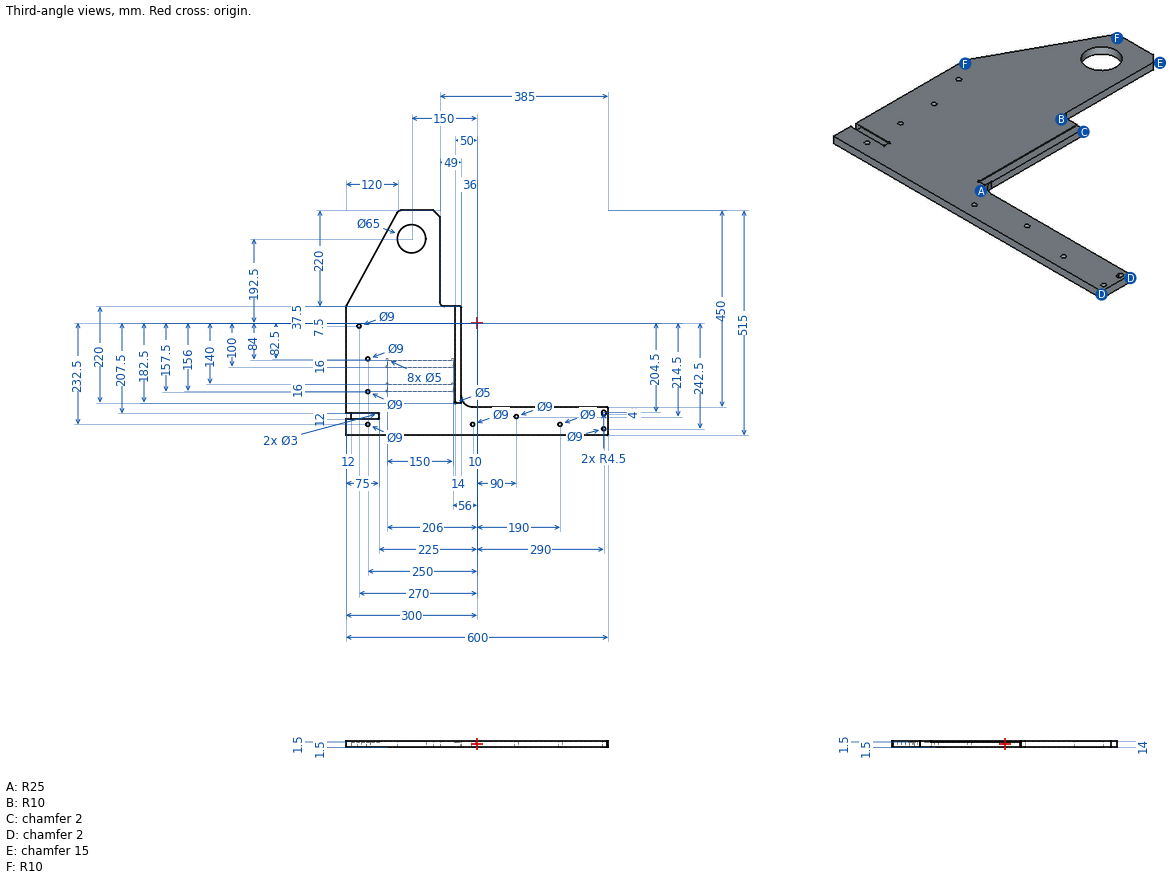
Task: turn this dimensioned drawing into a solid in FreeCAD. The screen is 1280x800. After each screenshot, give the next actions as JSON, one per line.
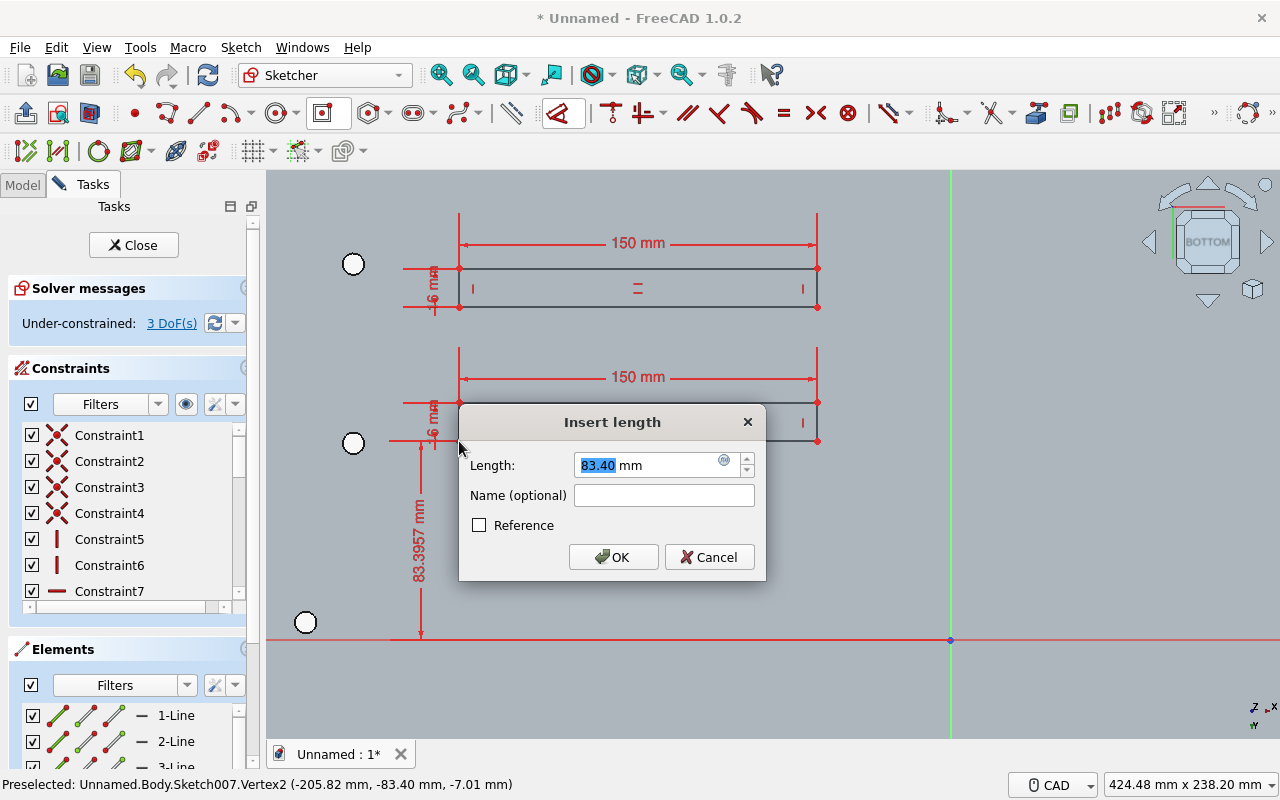
{"action": "type", "text": "84"}
{"action": "key", "text": "Return"}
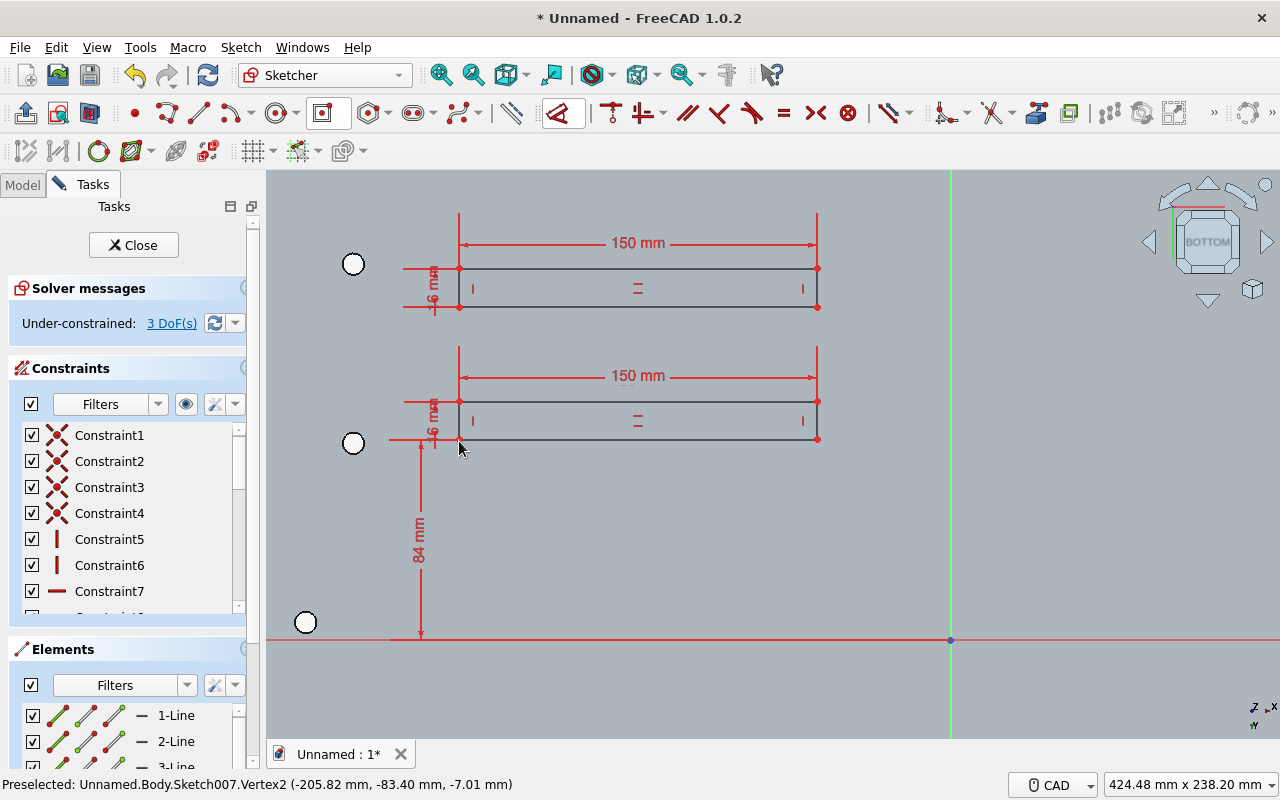
{"action": "left_click", "coordinate": [817, 440]}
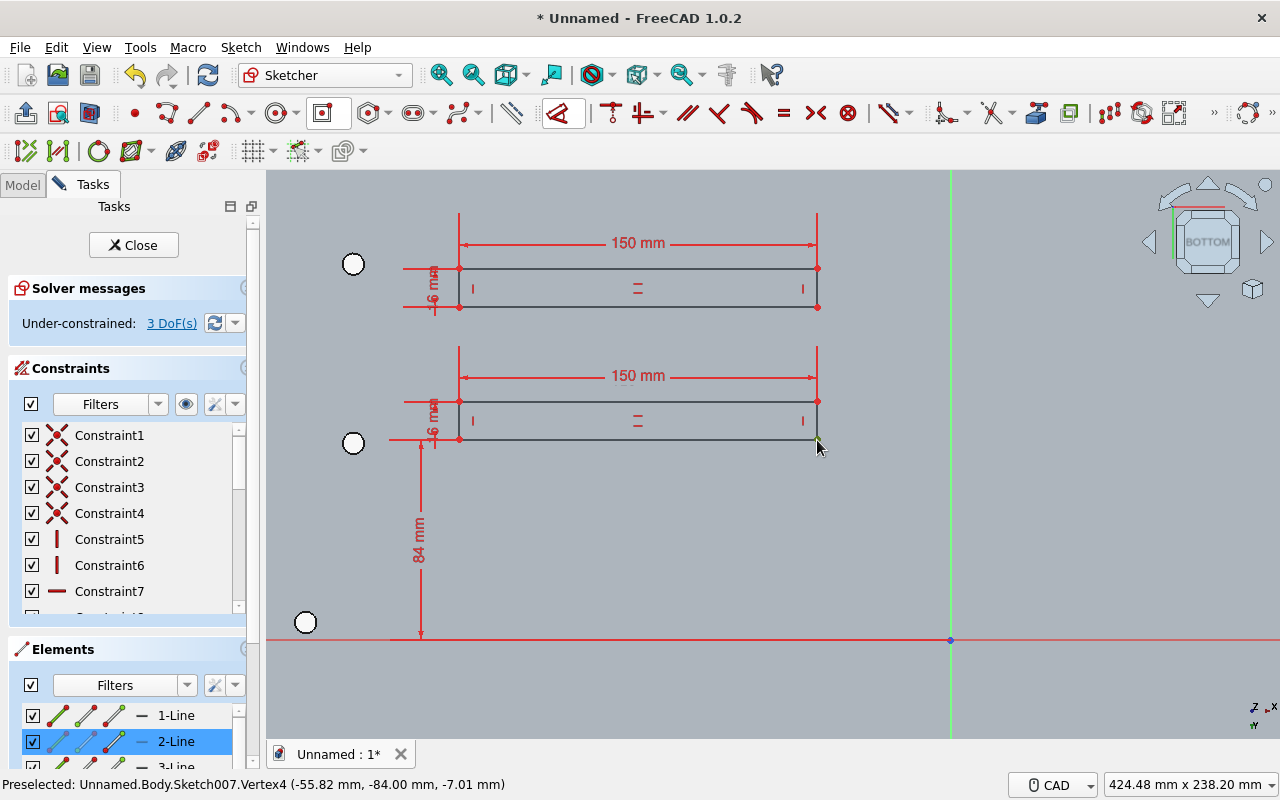
{"action": "left_click", "coordinate": [580, 114]}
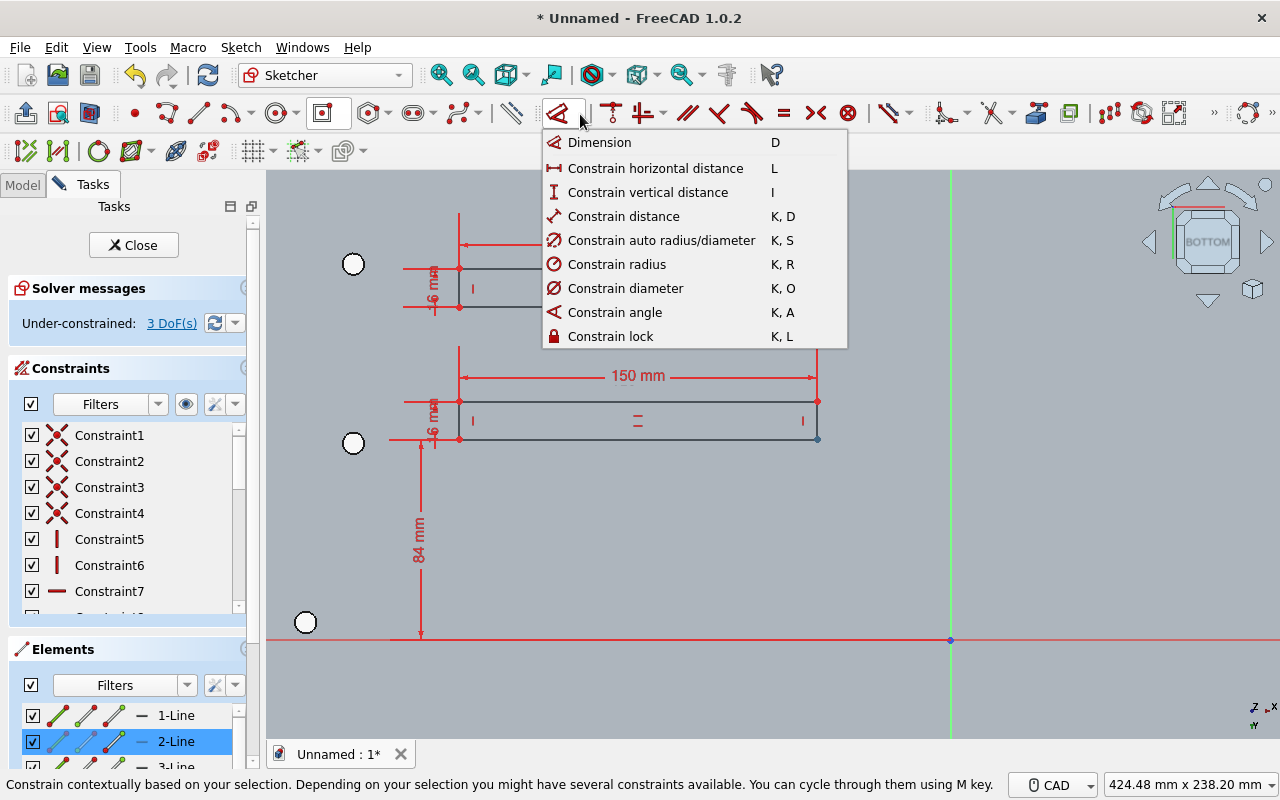
{"action": "left_click", "coordinate": [695, 168]}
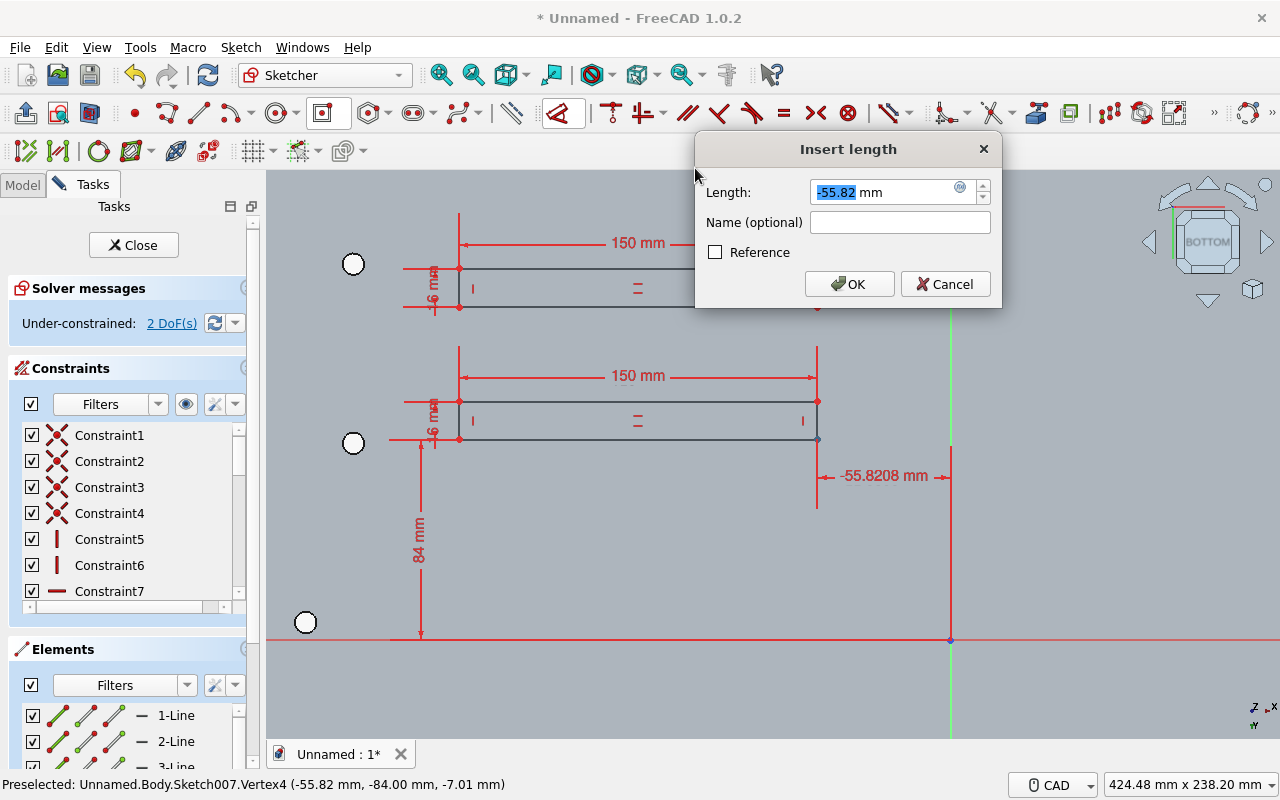
{"action": "type", "text": "-56"}
{"action": "key", "text": "Return"}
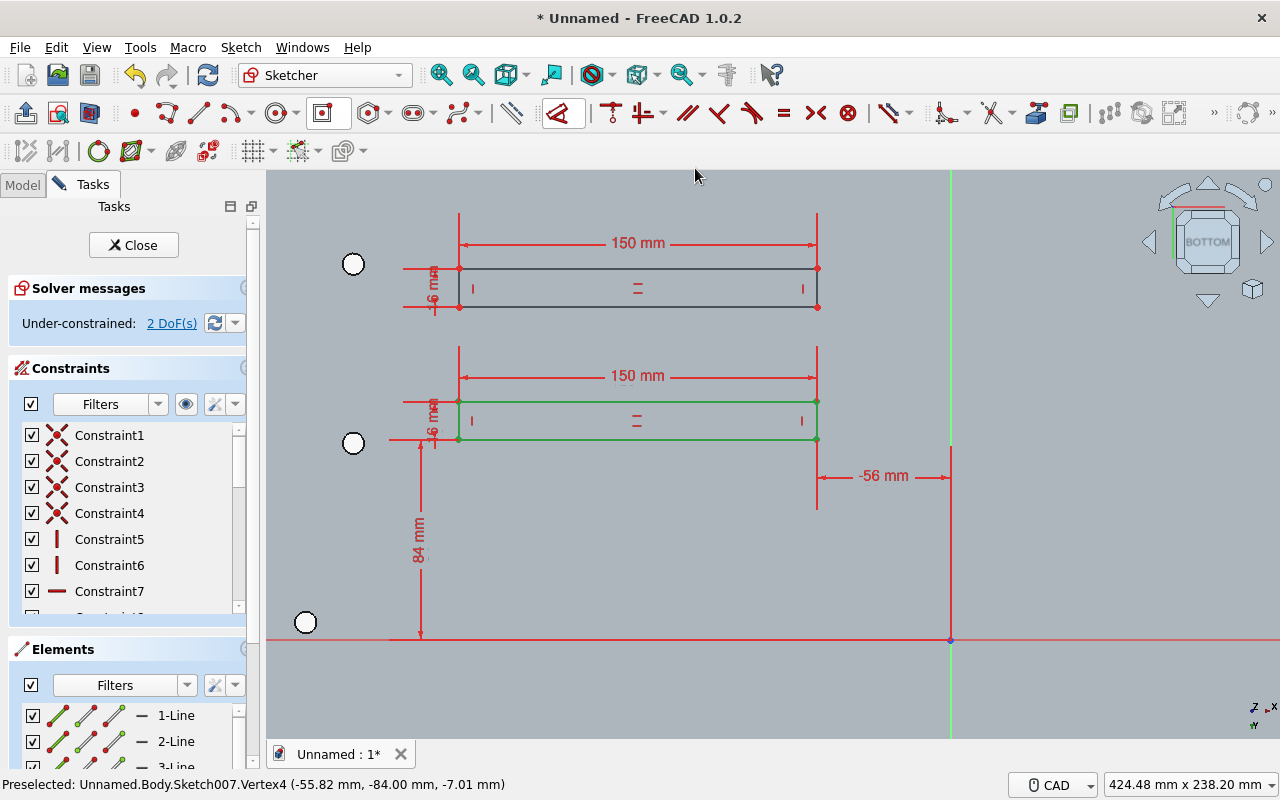
{"action": "left_click", "coordinate": [817, 307]}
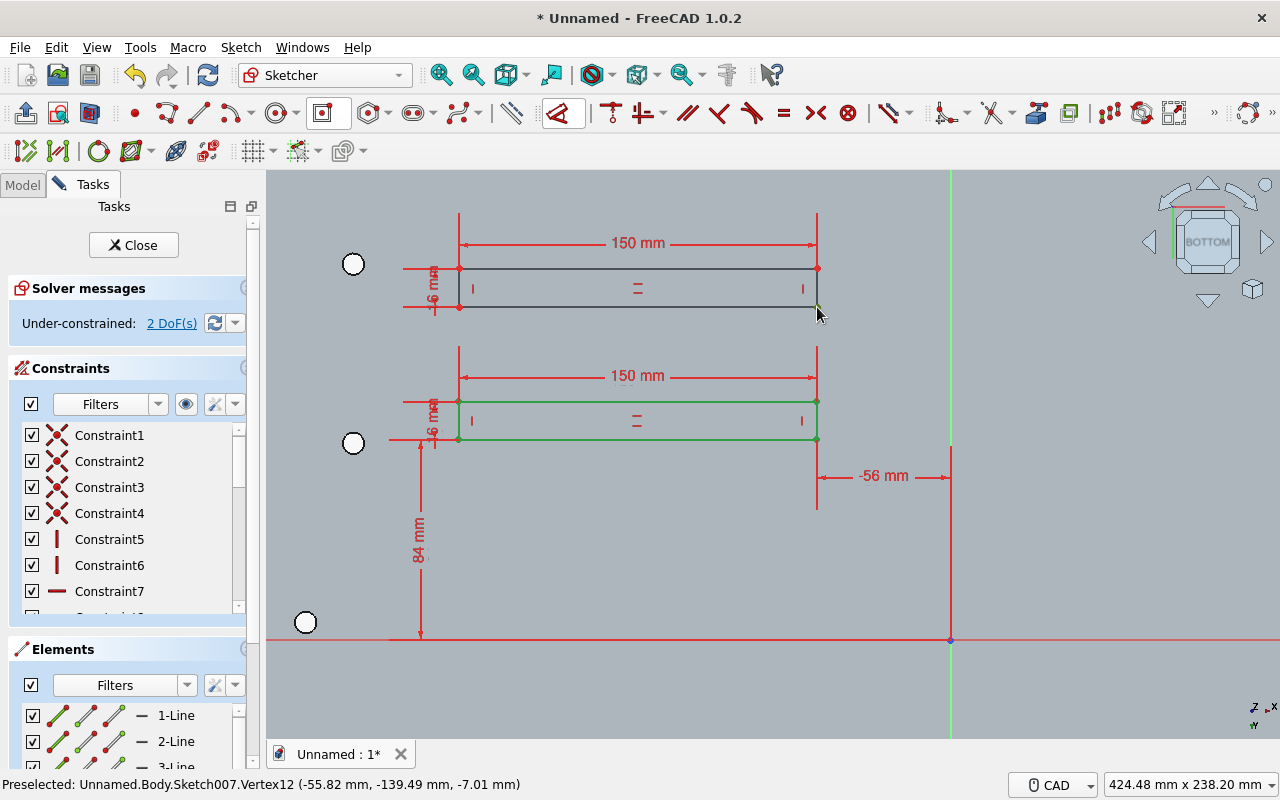
{"action": "left_click", "coordinate": [580, 114]}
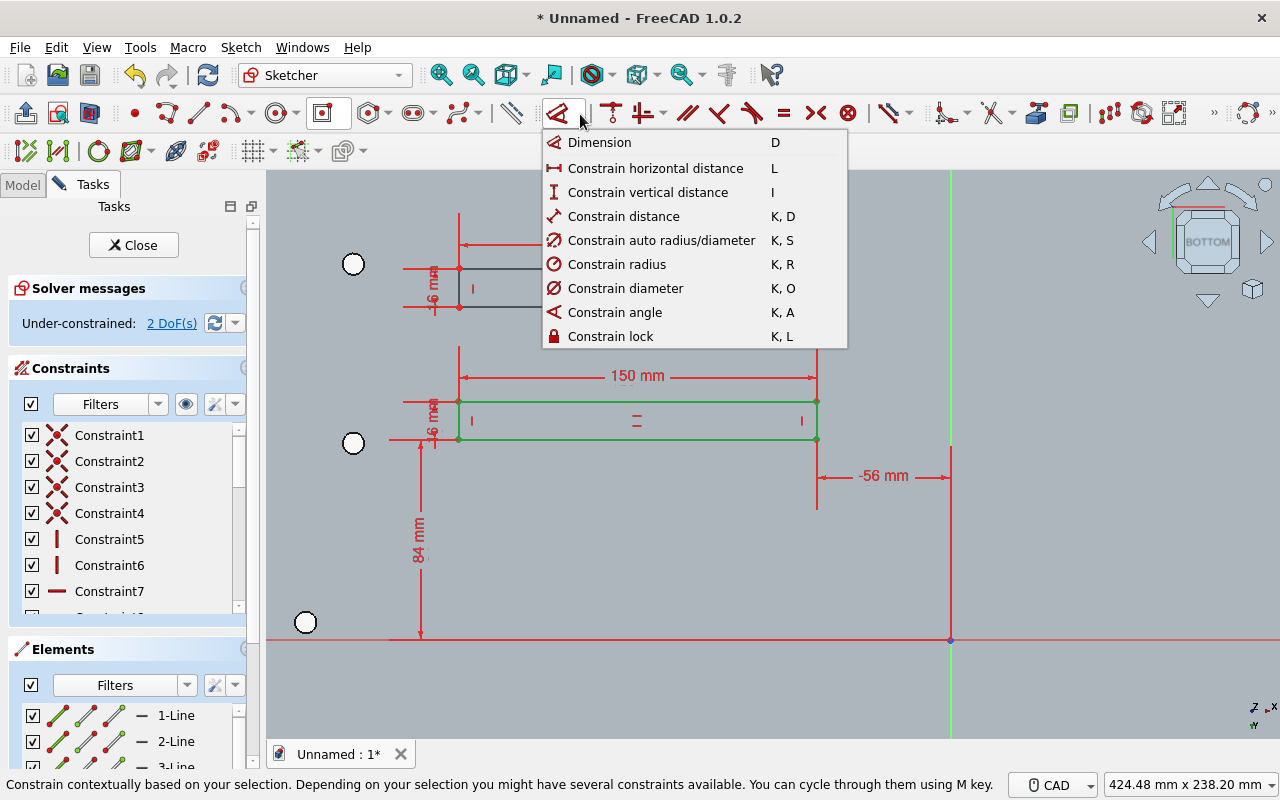
{"action": "left_click", "coordinate": [695, 168]}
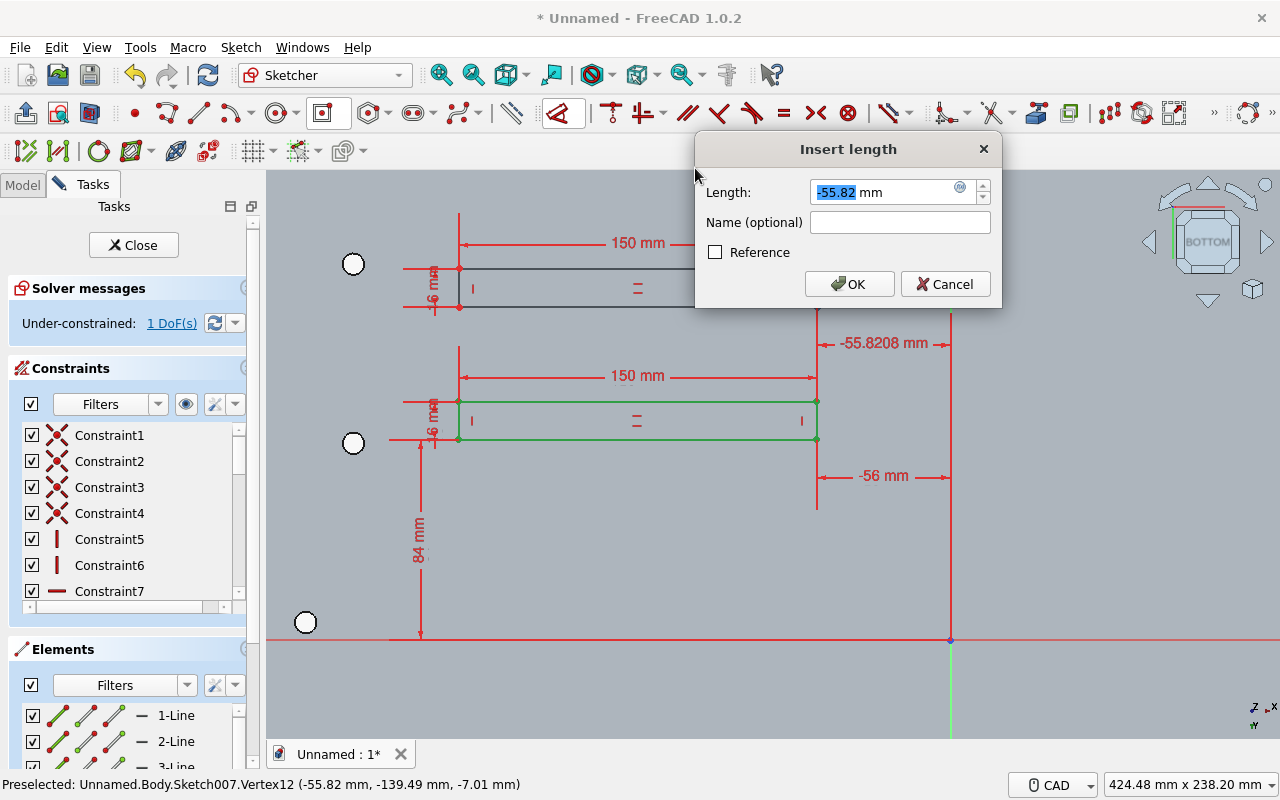
{"action": "type", "text": "-56"}
{"action": "key", "text": "Return"}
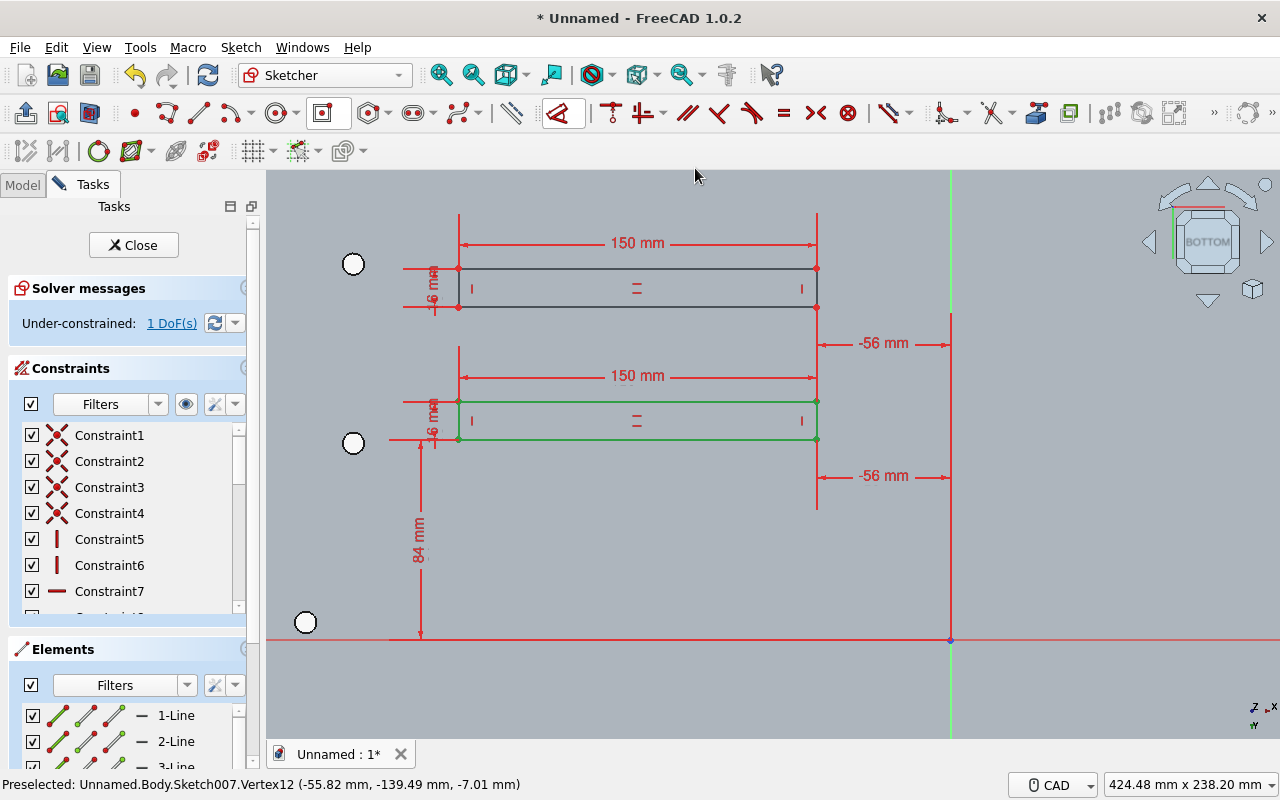
{"action": "left_click", "coordinate": [459, 269]}